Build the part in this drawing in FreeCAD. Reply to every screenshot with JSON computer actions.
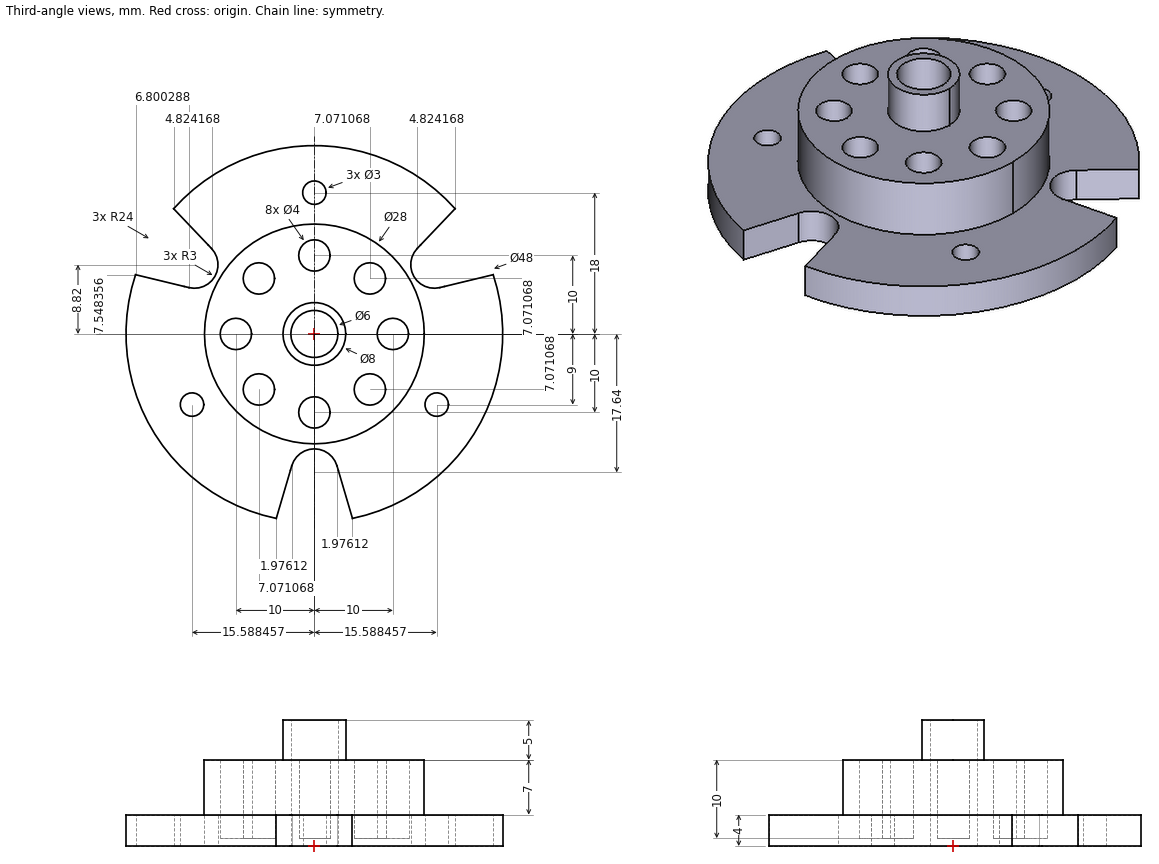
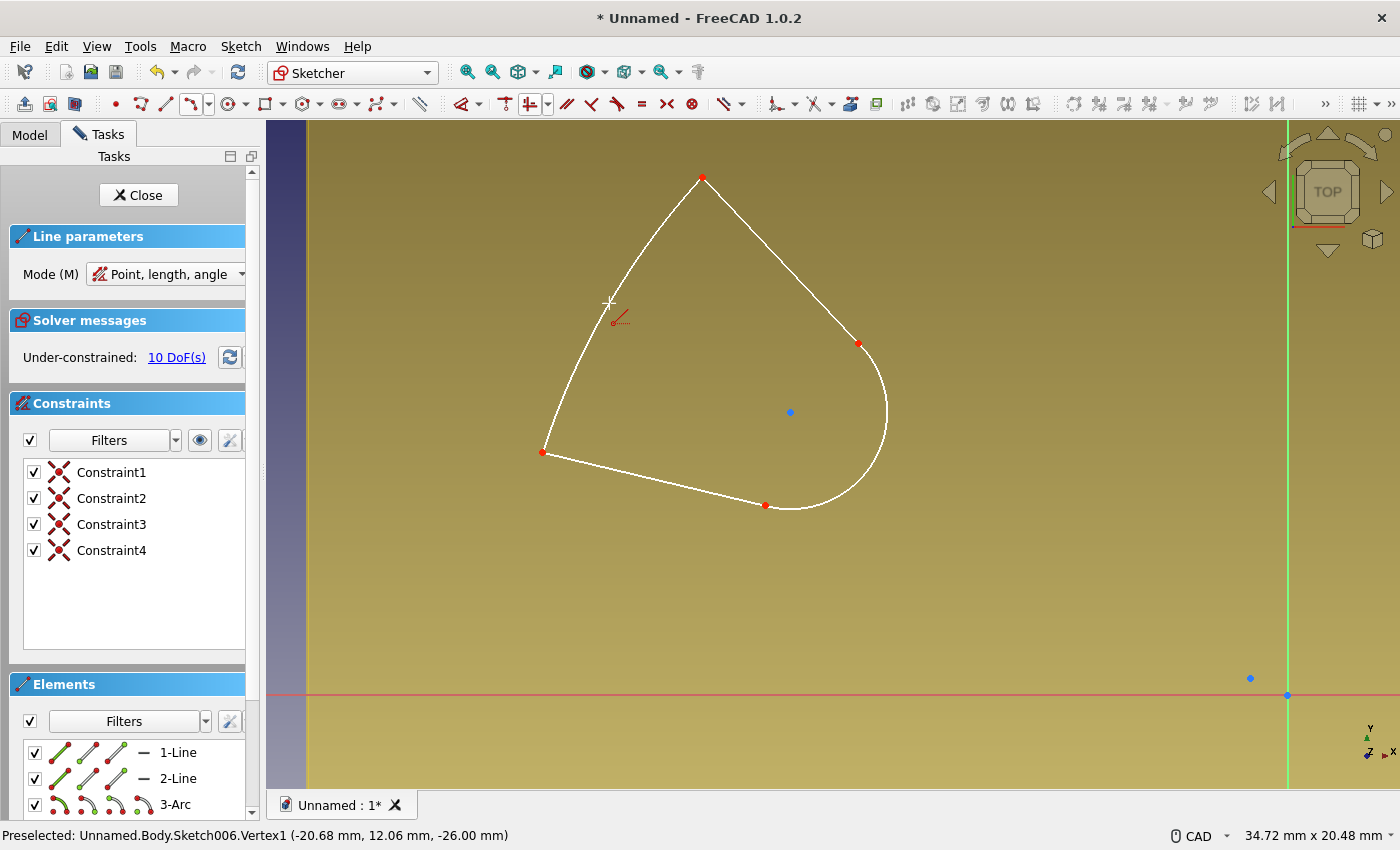
{"action": "scroll", "coordinate": [539, 294], "scroll_direction": "down", "scroll_amount": 6}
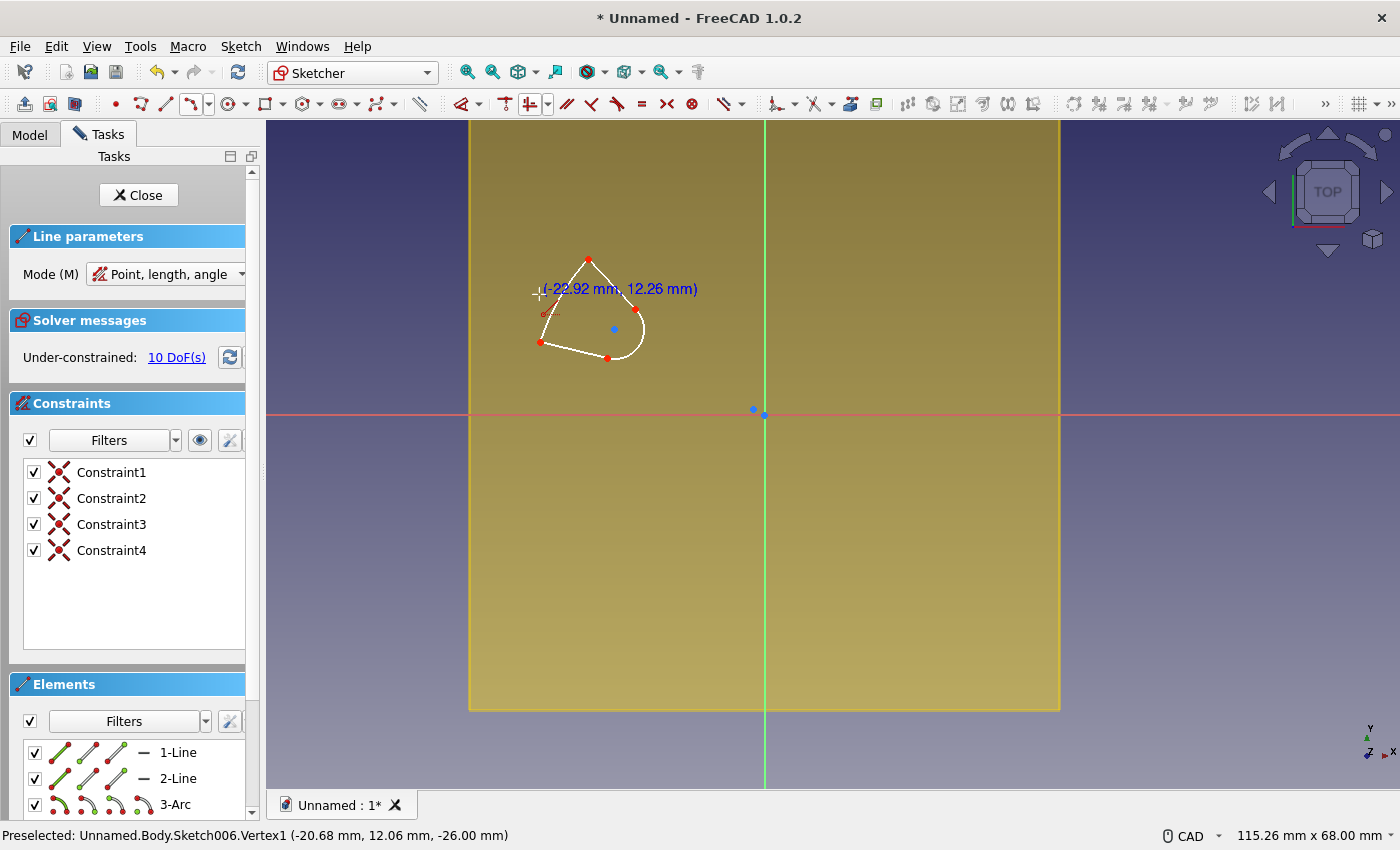
{"action": "left_click", "coordinate": [941, 258]}
{"action": "left_click", "coordinate": [894, 308]}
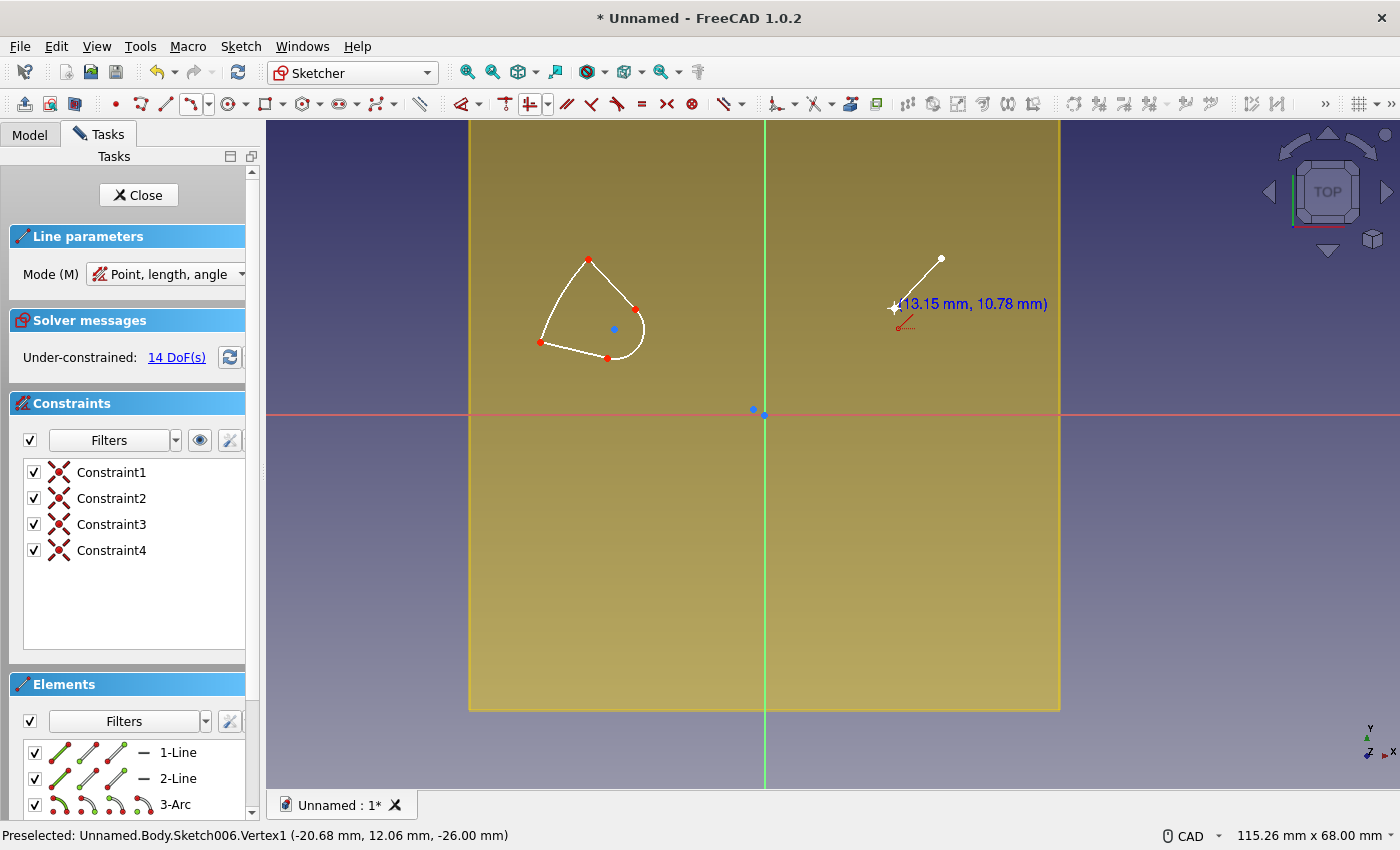
{"action": "left_click", "coordinate": [922, 357]}
{"action": "left_click", "coordinate": [989, 341]}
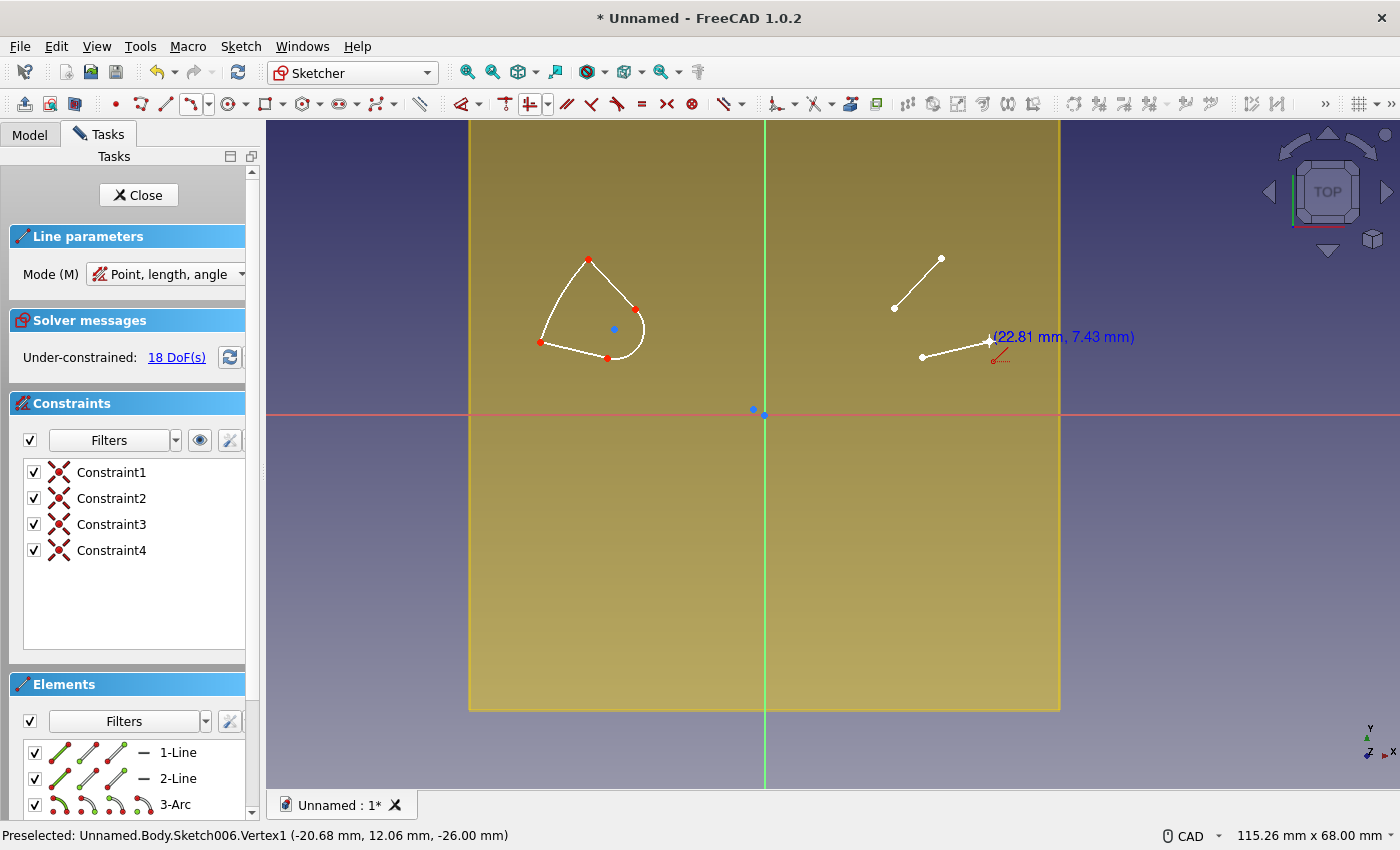
{"action": "left_click", "coordinate": [190, 104]}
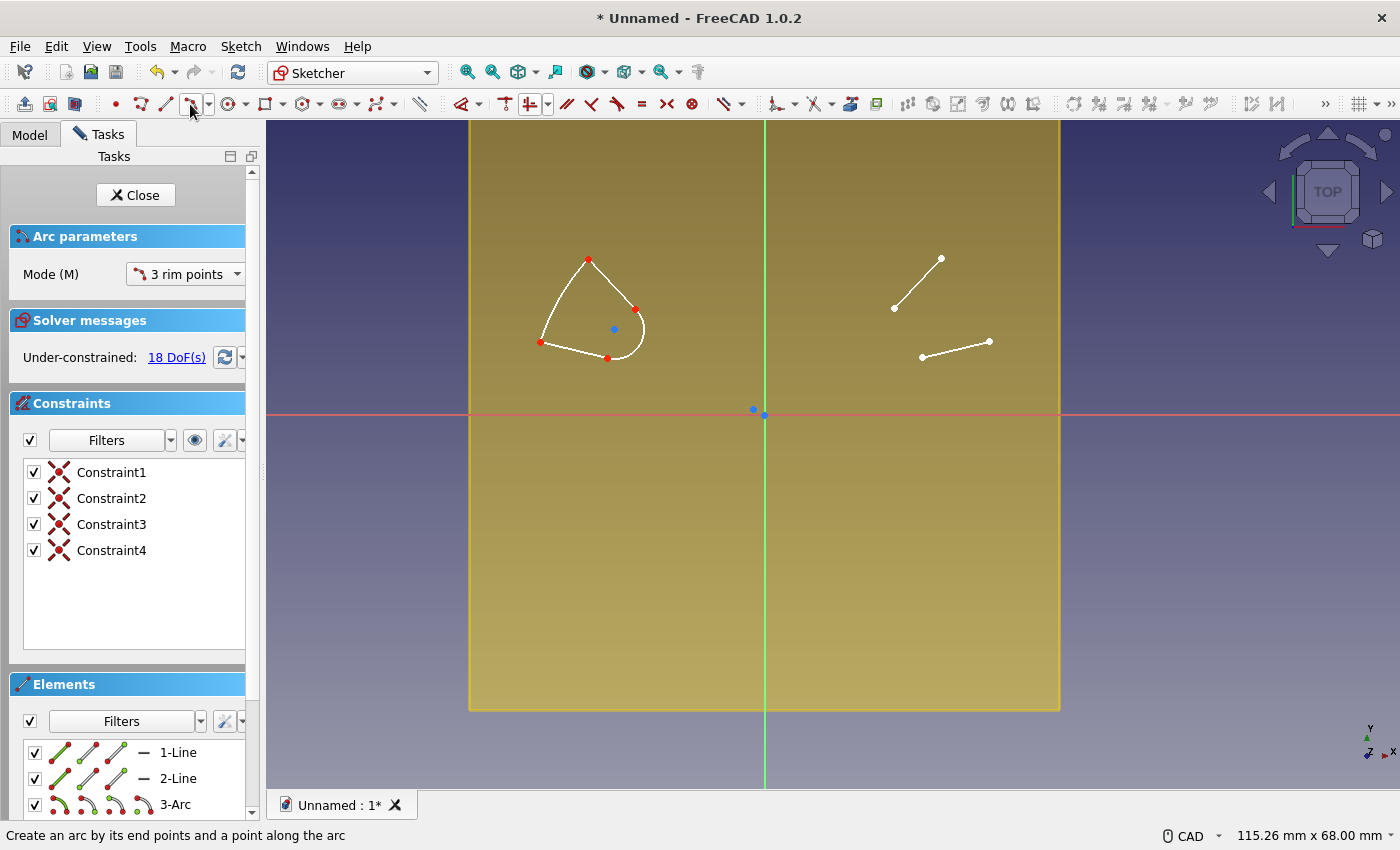
{"action": "left_click", "coordinate": [894, 309]}
{"action": "left_click", "coordinate": [922, 358]}
{"action": "left_click", "coordinate": [889, 343]}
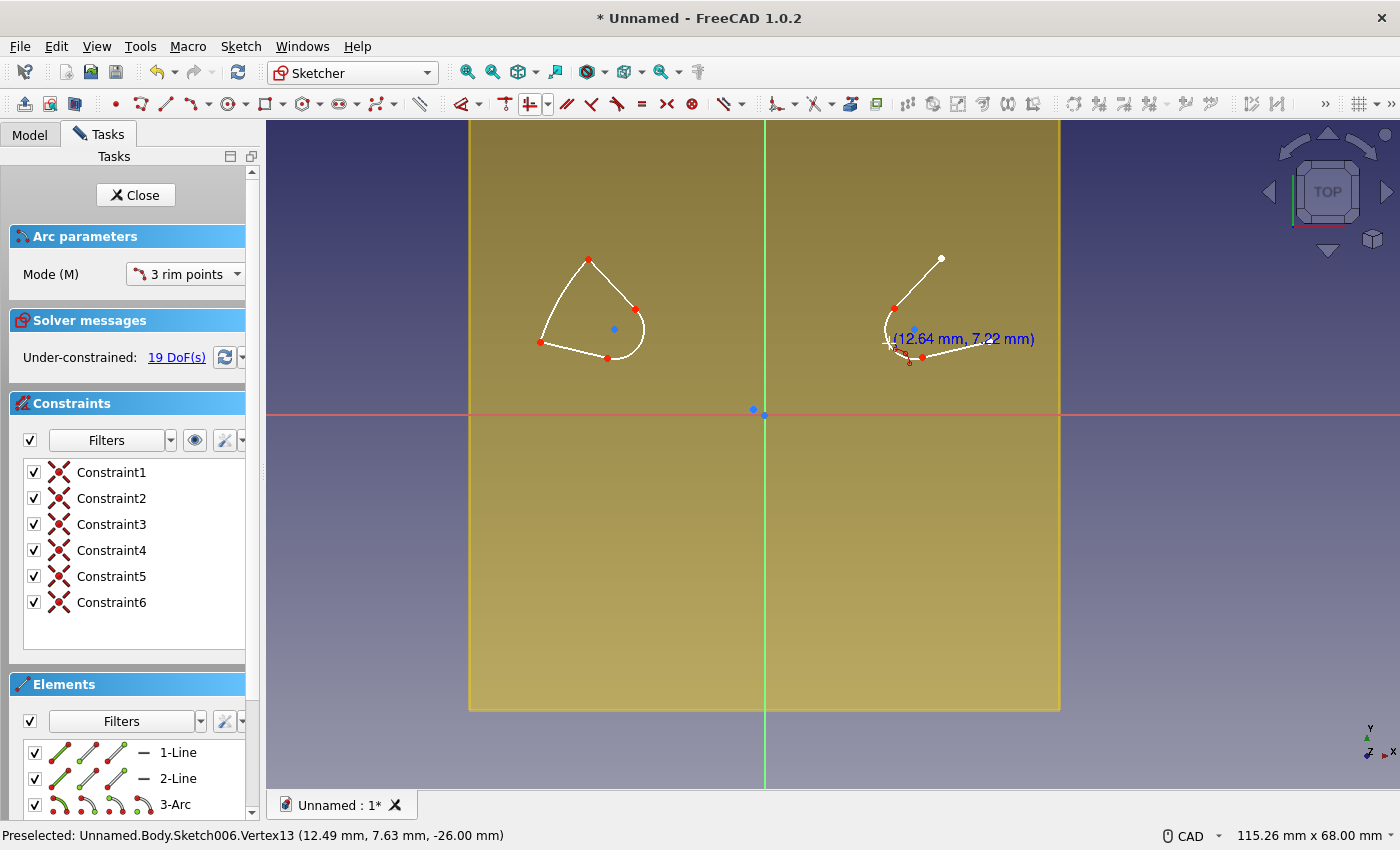
{"action": "left_click", "coordinate": [989, 342]}
{"action": "left_click", "coordinate": [941, 259]}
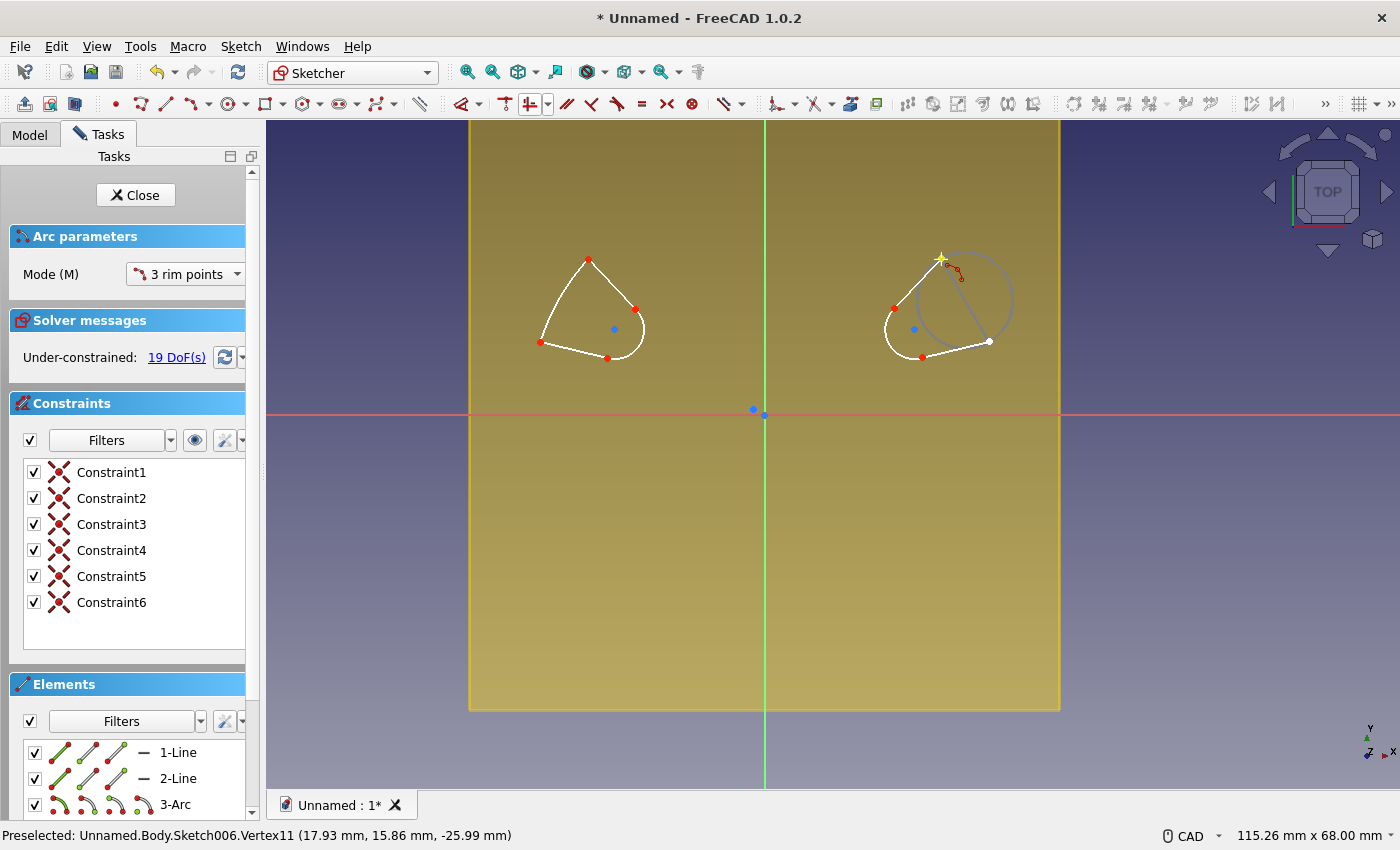
{"action": "scroll", "coordinate": [969, 297], "scroll_direction": "up", "scroll_amount": 6}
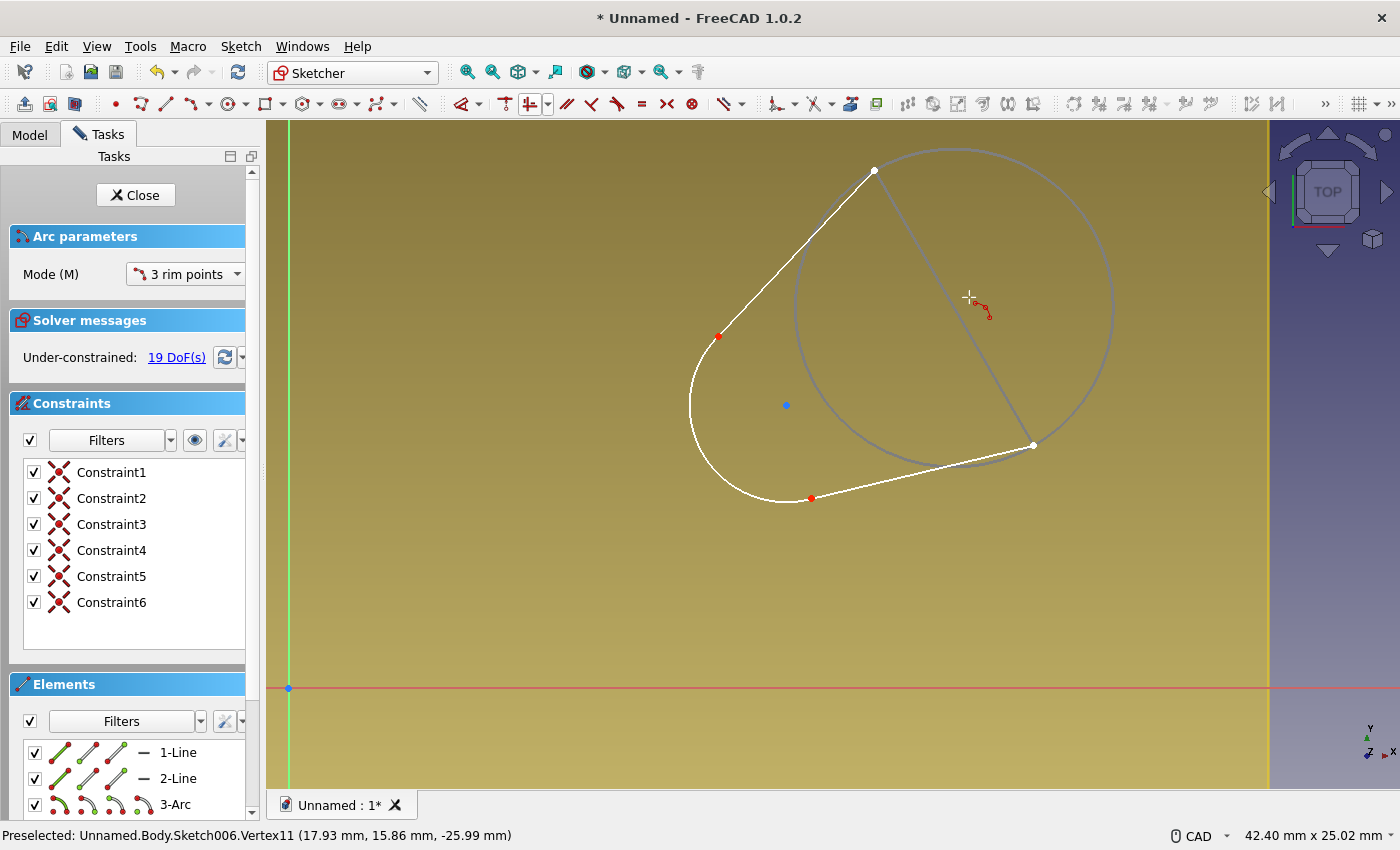
{"action": "left_click", "coordinate": [968, 296]}